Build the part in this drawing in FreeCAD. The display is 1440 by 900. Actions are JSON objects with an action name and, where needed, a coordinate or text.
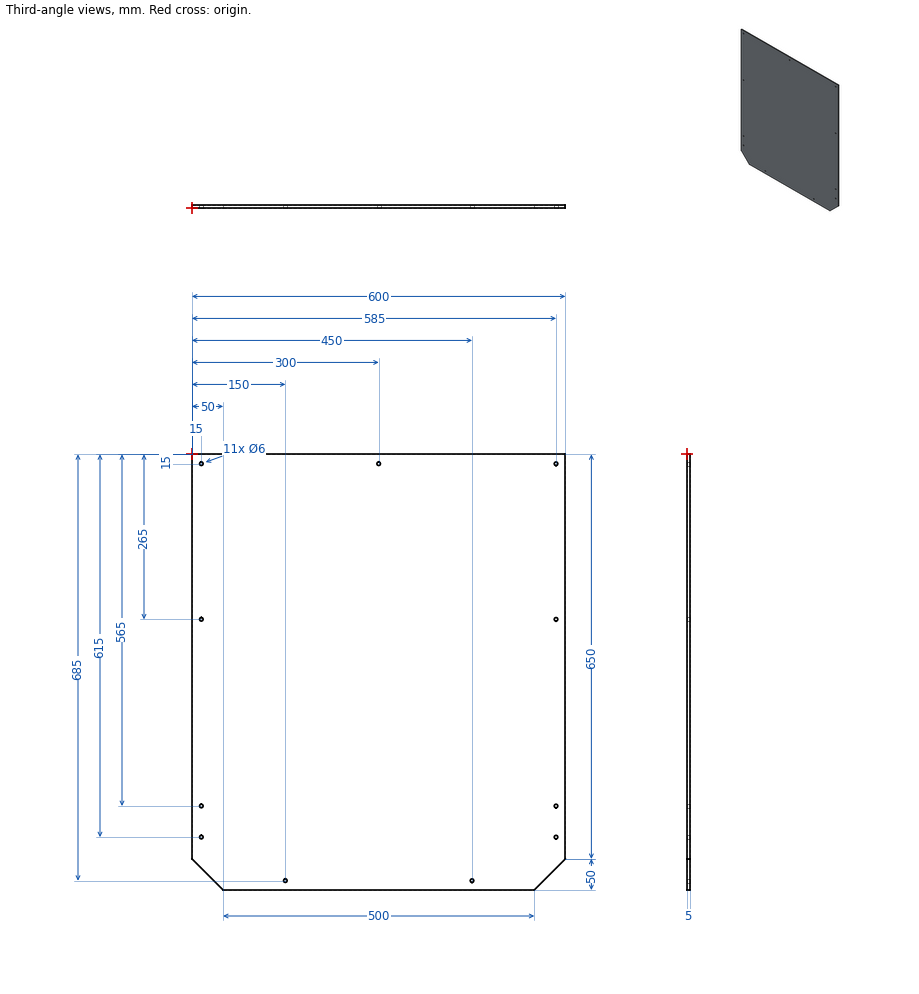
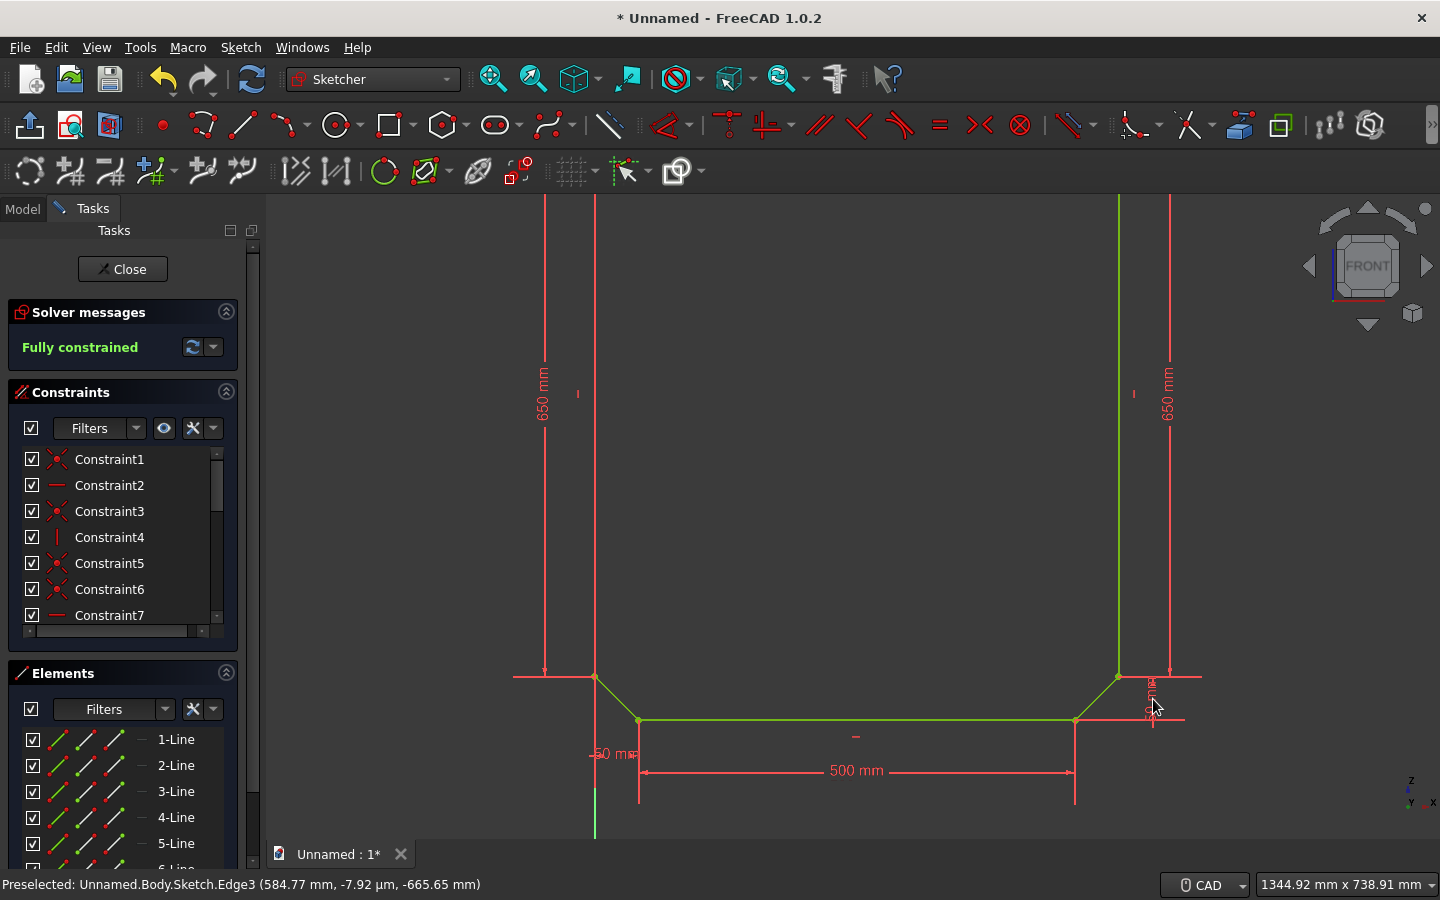
{"action": "left_click", "coordinate": [123, 269]}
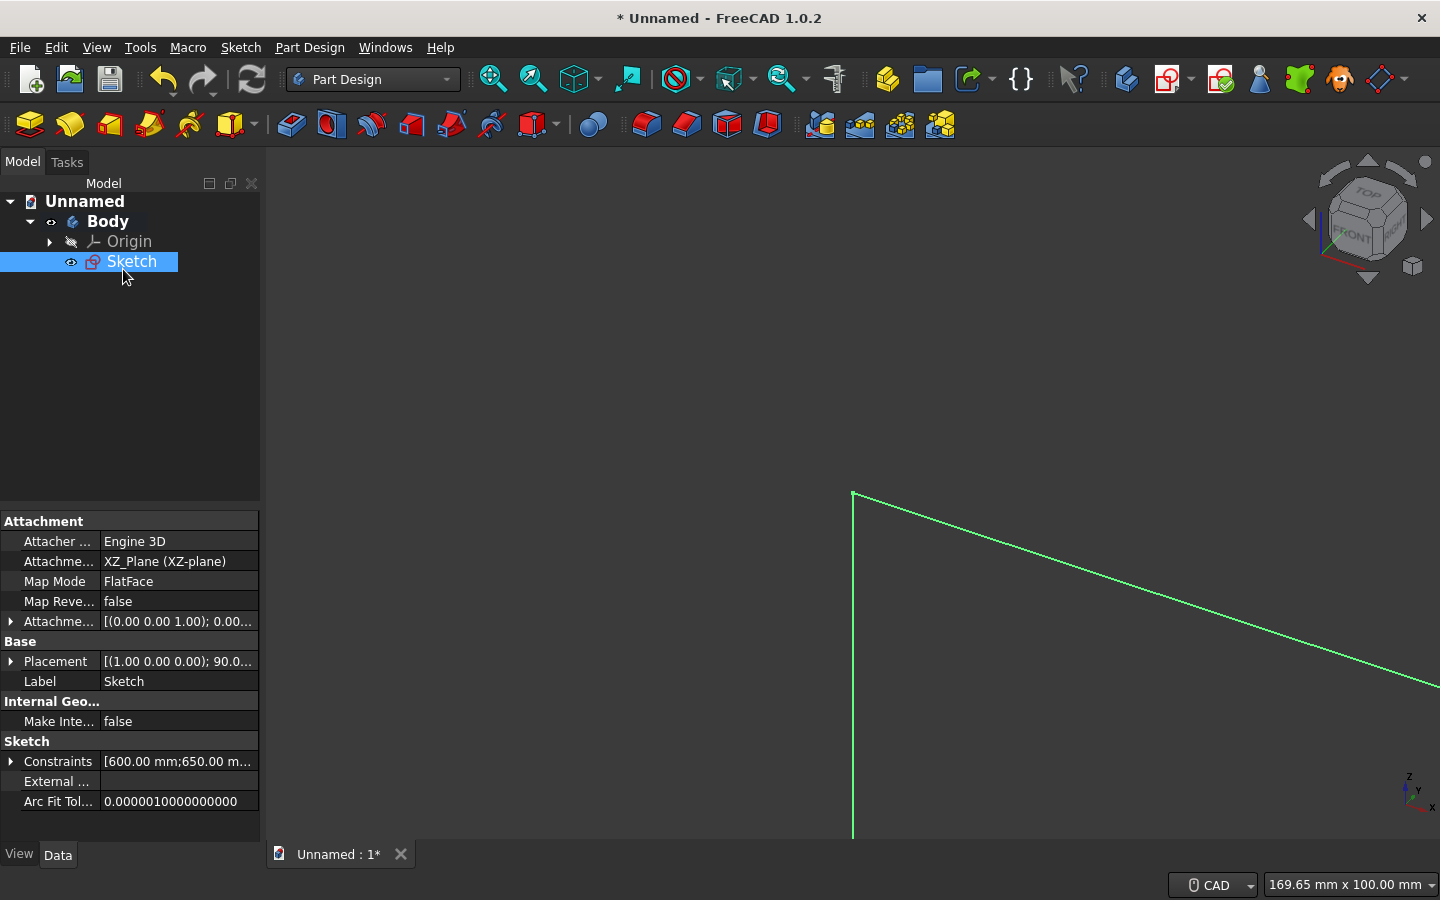
{"action": "left_click", "coordinate": [30, 124]}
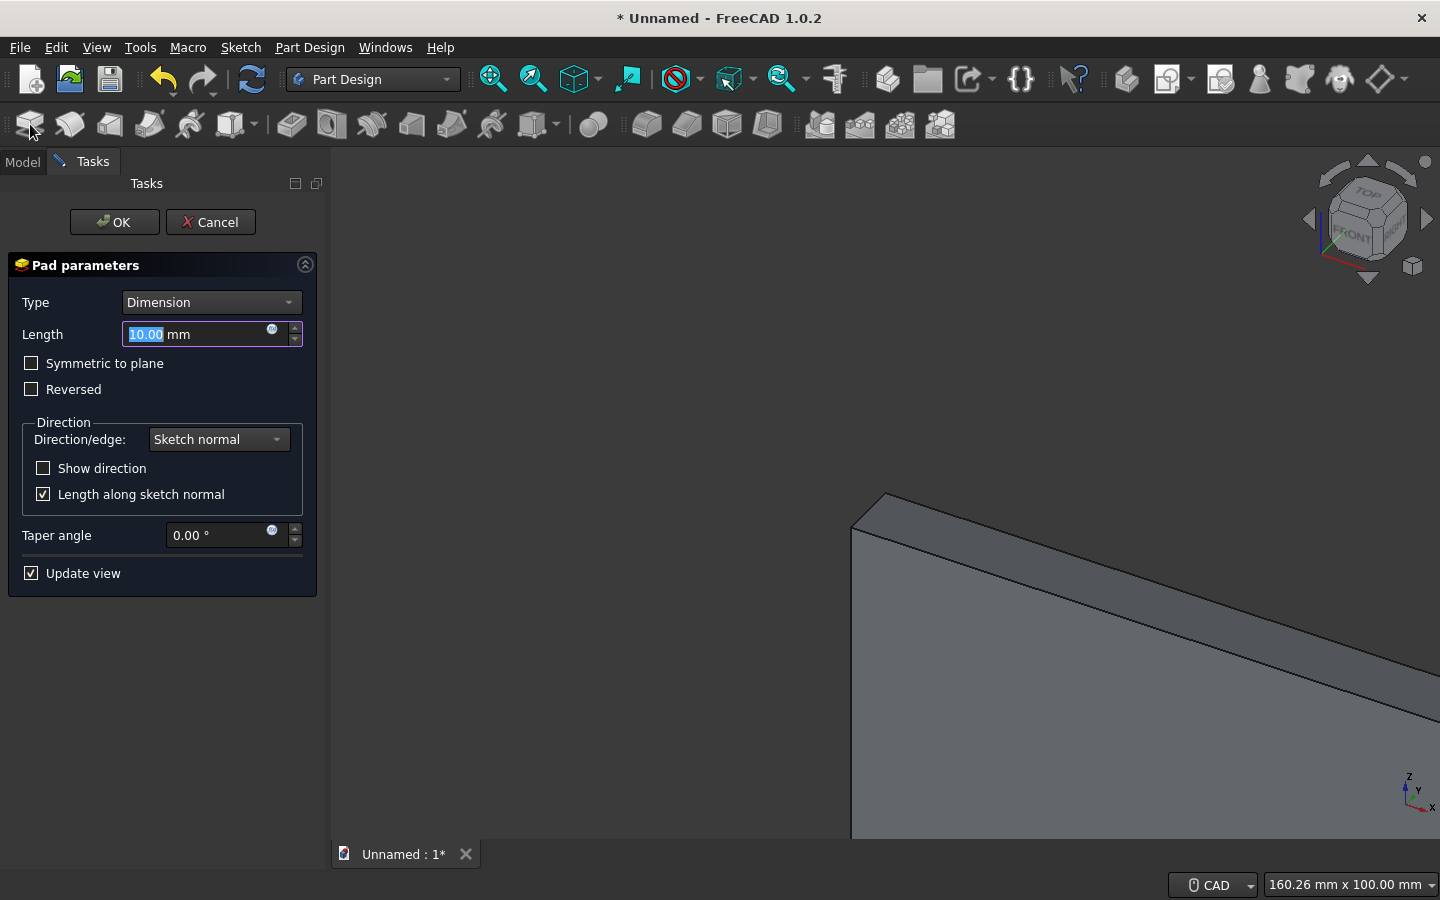
{"action": "type", "text": "5"}
{"action": "key", "text": "Tab"}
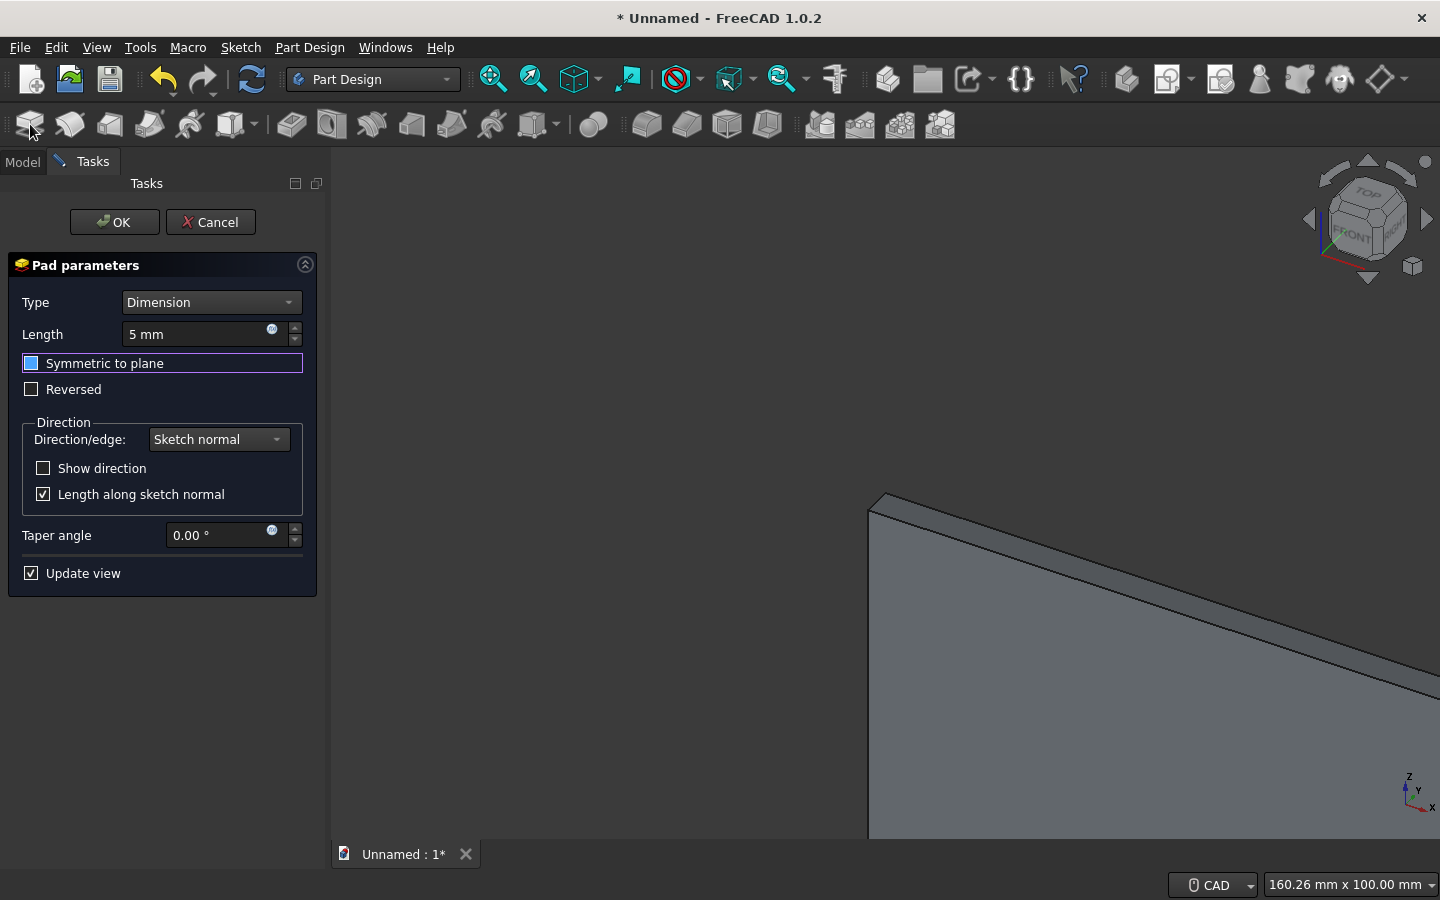
{"action": "left_click", "coordinate": [30, 389]}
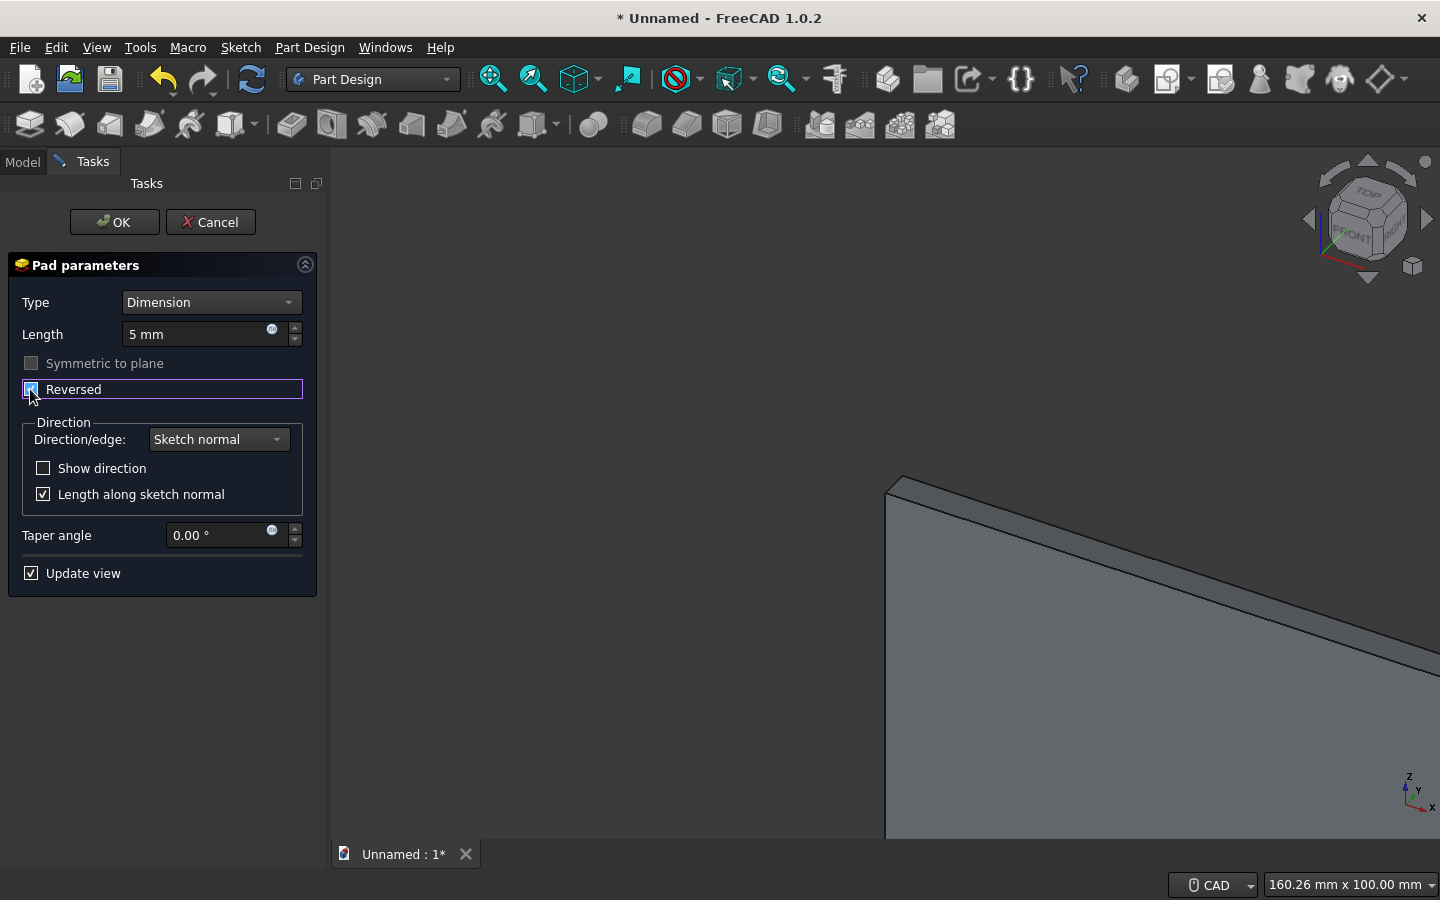
{"action": "left_click", "coordinate": [115, 222]}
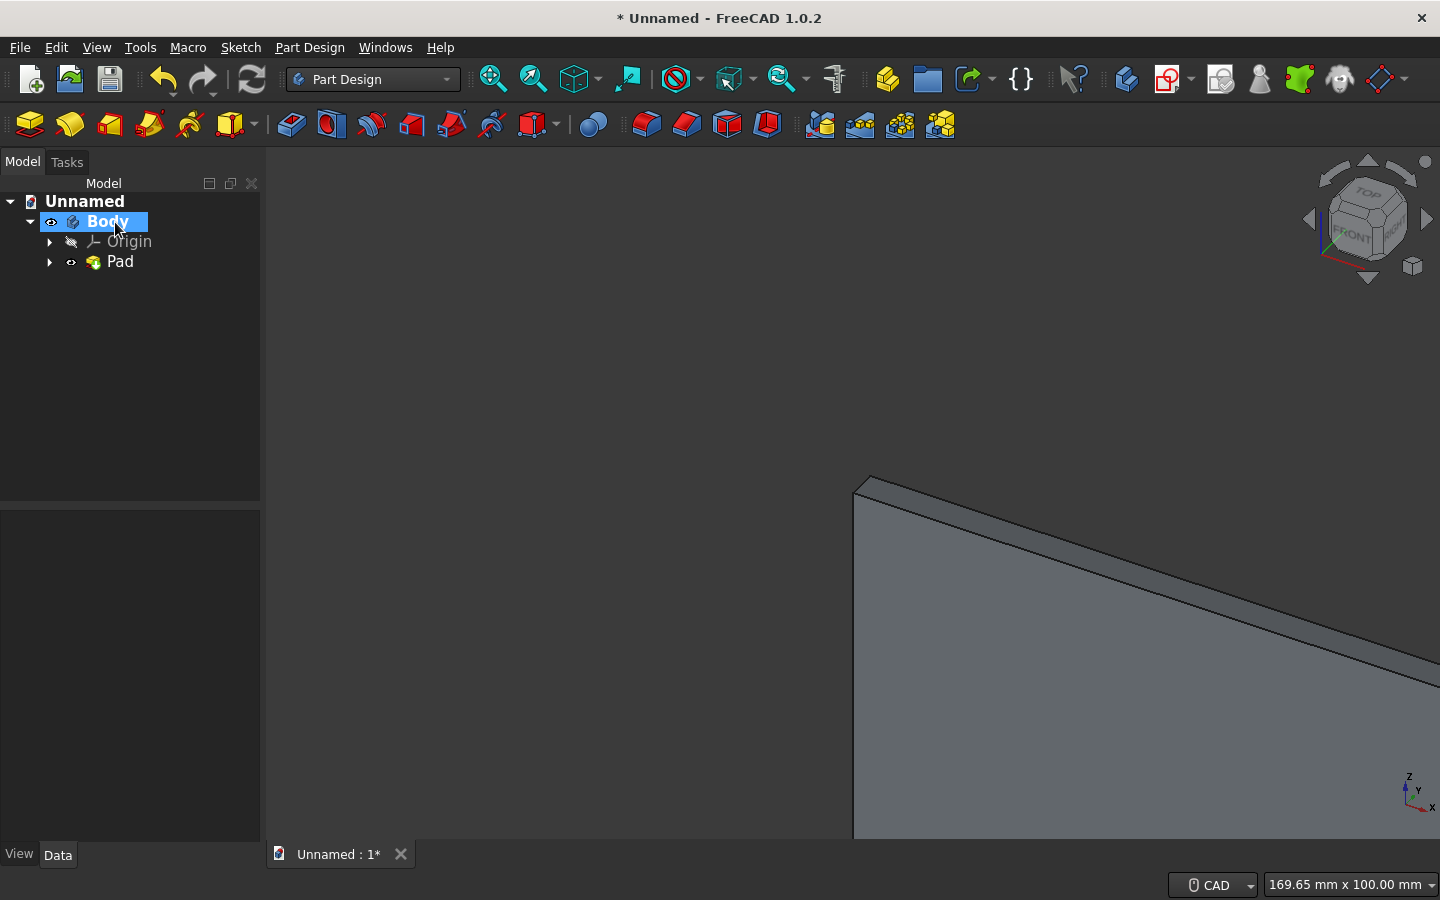
{"action": "key", "text": "v f"}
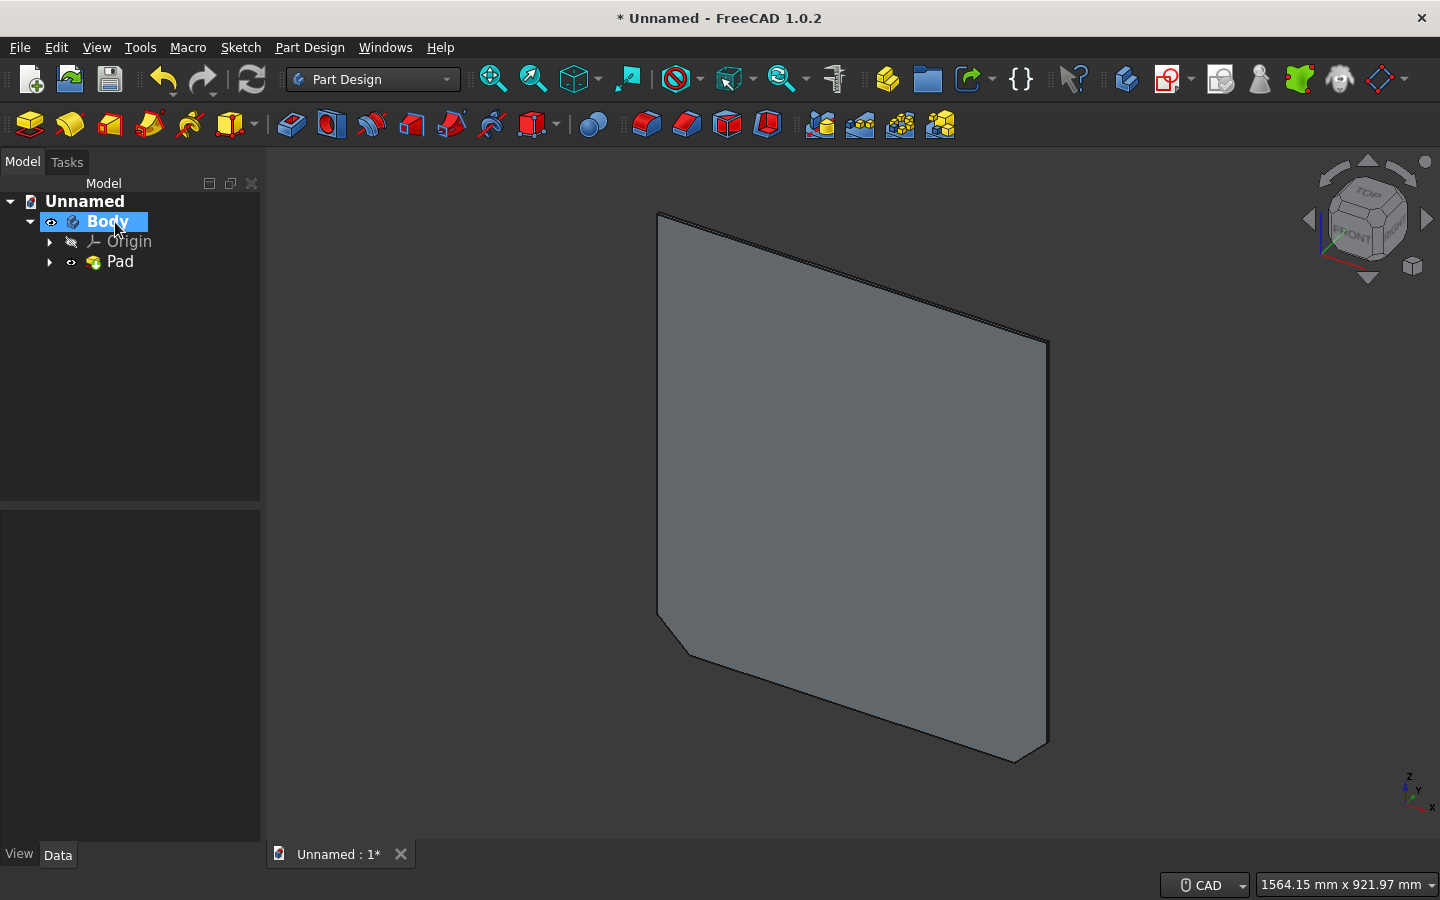
{"action": "key", "text": "4"}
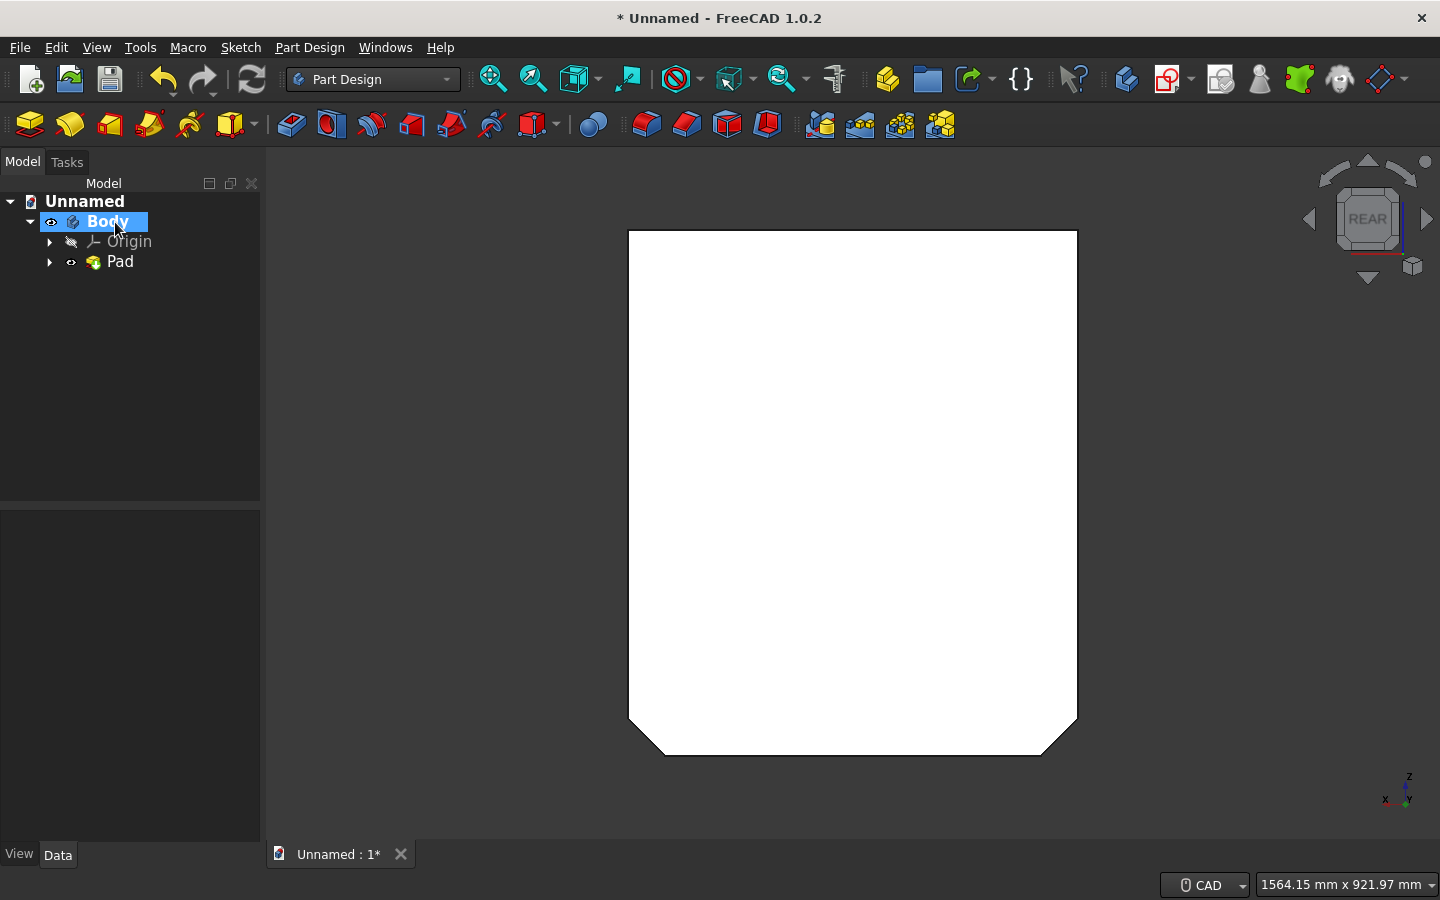
{"action": "left_click", "coordinate": [853, 492]}